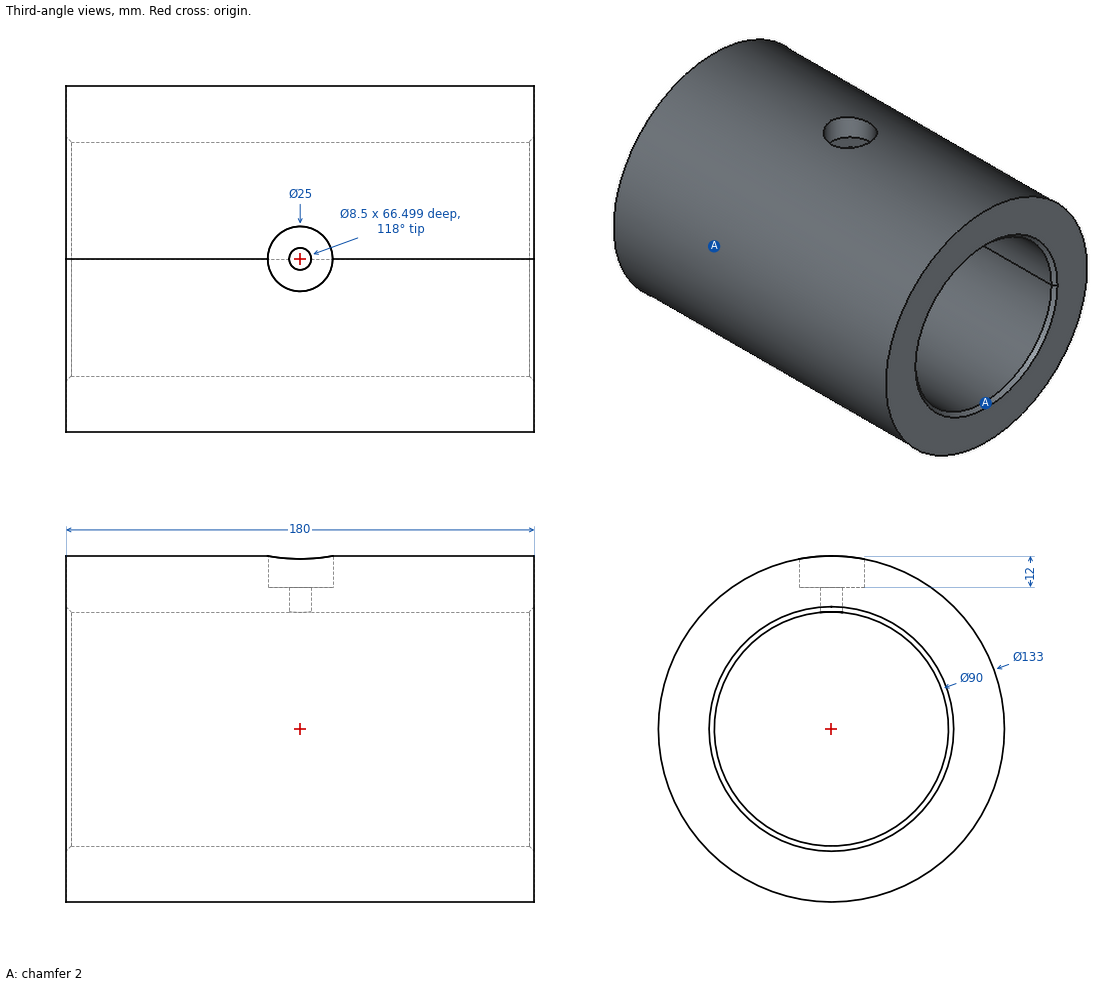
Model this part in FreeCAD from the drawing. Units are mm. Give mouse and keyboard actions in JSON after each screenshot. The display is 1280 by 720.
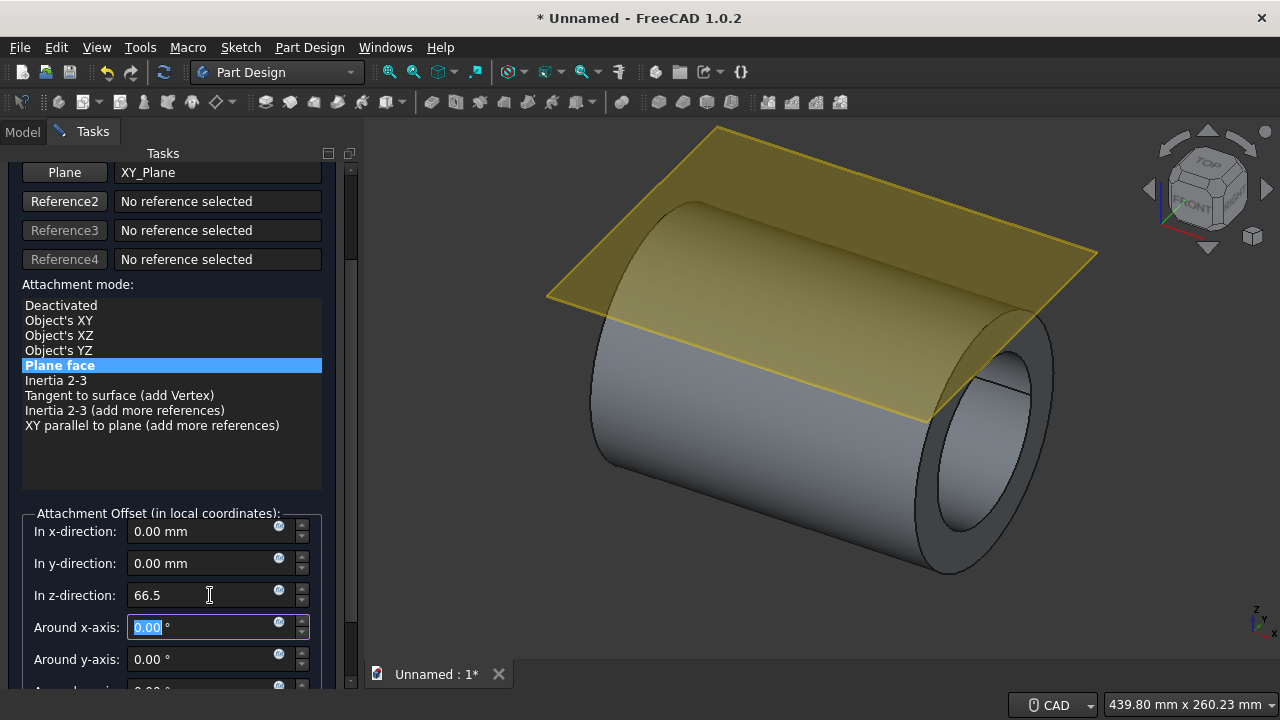
{"action": "scroll", "coordinate": [351, 426], "scroll_direction": "up", "scroll_amount": 3}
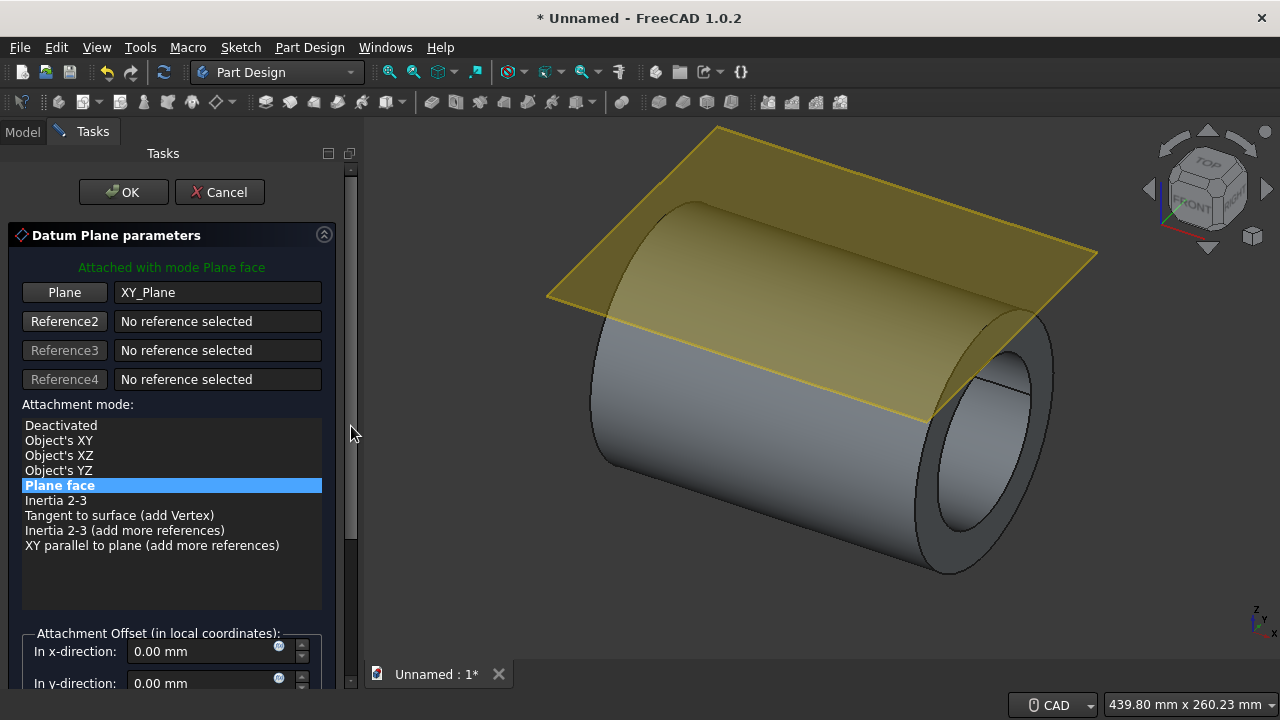
{"action": "left_click", "coordinate": [124, 192]}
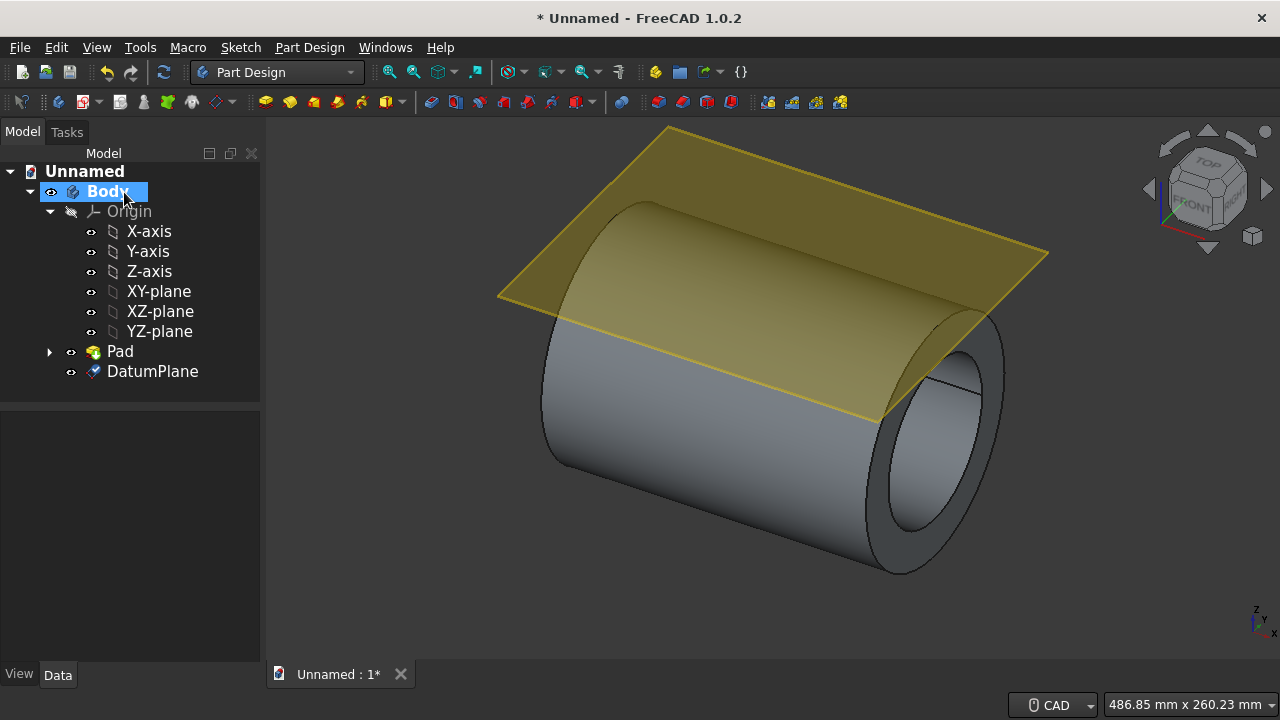
{"action": "left_click", "coordinate": [116, 372]}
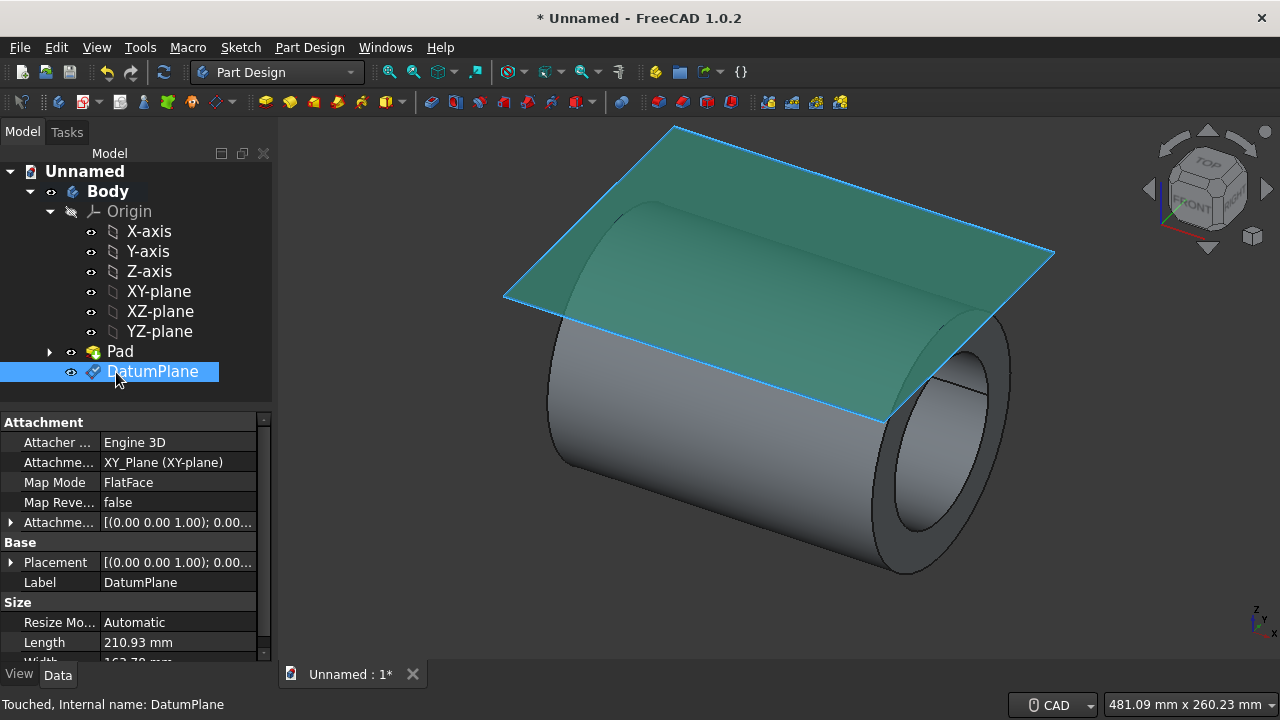
{"action": "left_click", "coordinate": [84, 102]}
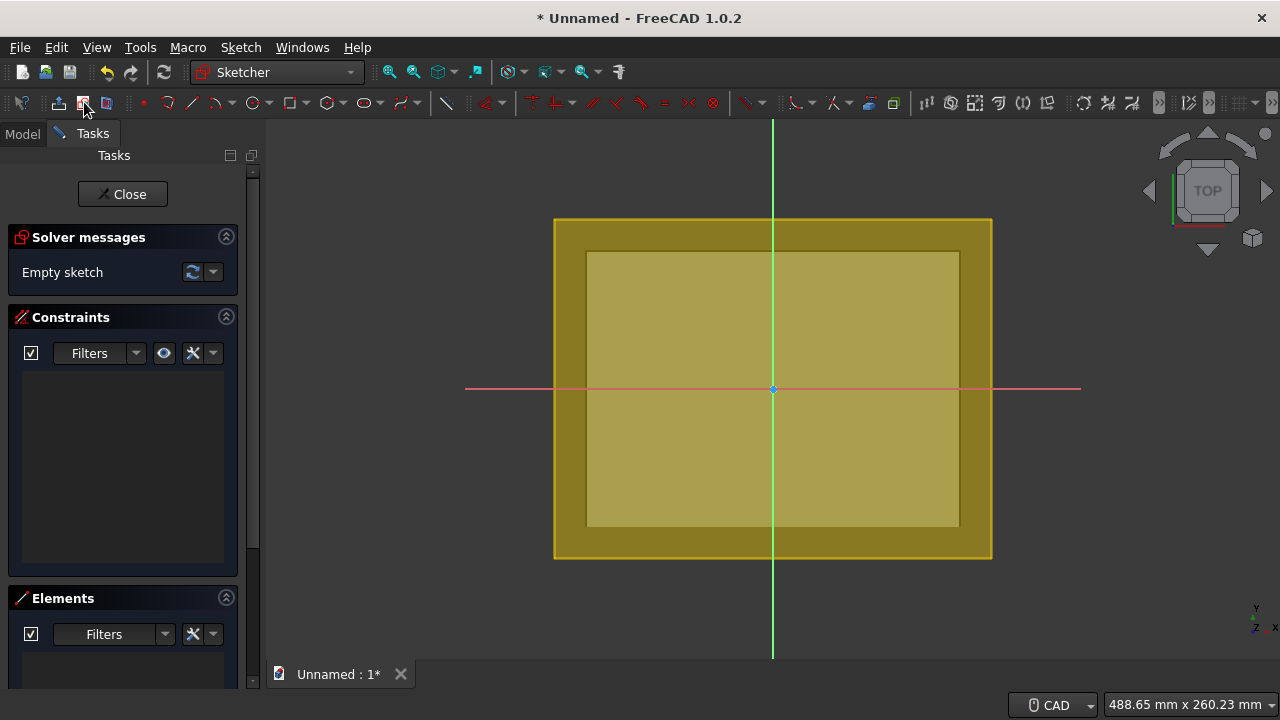
{"action": "scroll", "coordinate": [777, 389], "scroll_direction": "up", "scroll_amount": 15}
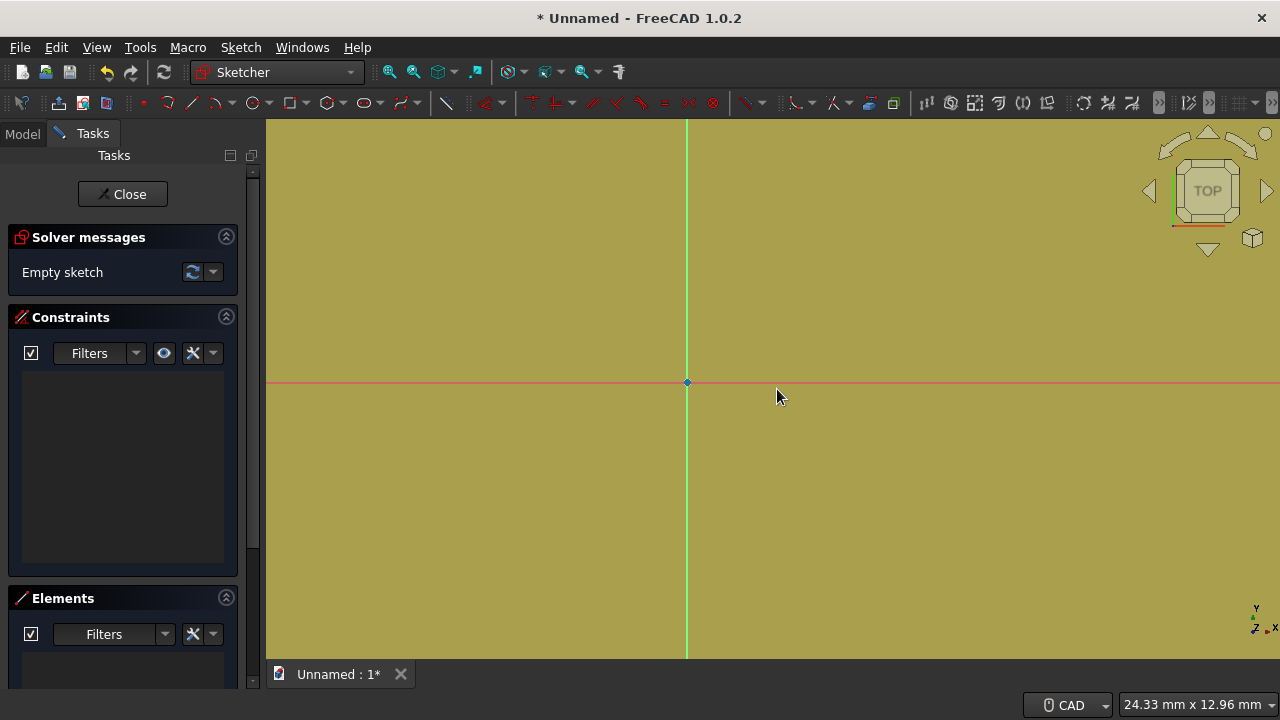
{"action": "left_click", "coordinate": [254, 104]}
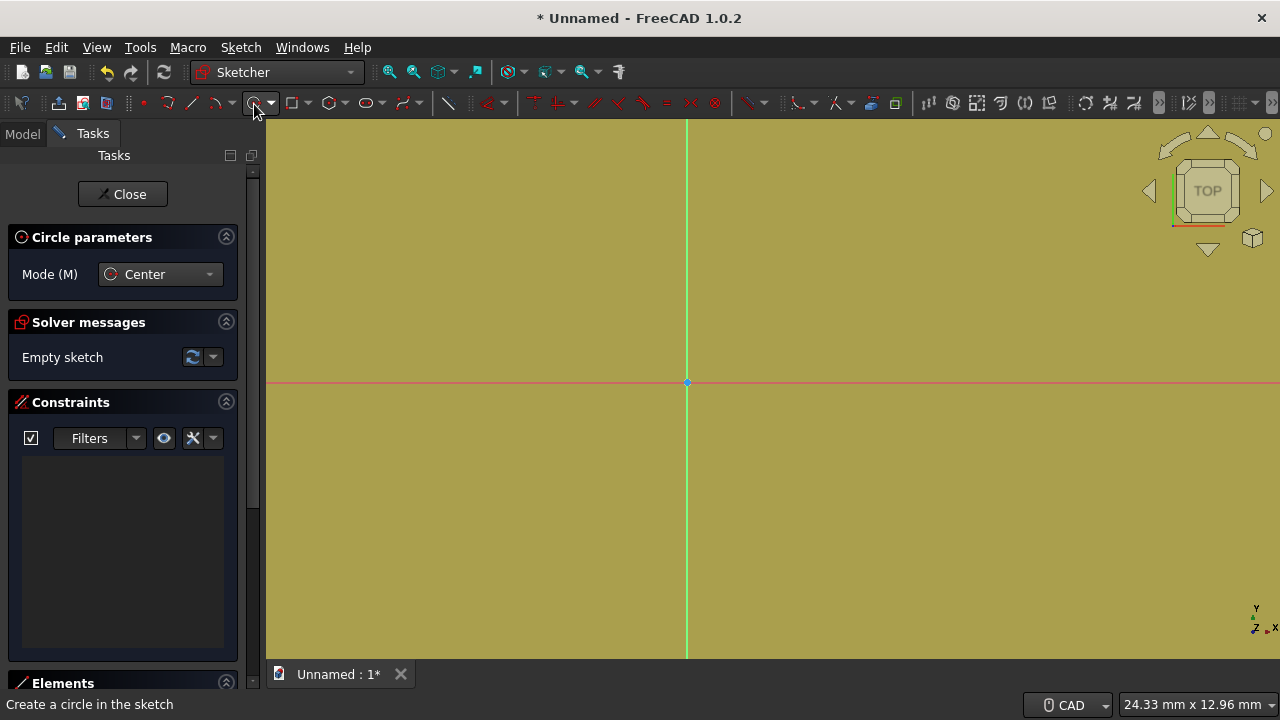
{"action": "left_click", "coordinate": [687, 383]}
{"action": "mouse_move", "coordinate": [812, 257]}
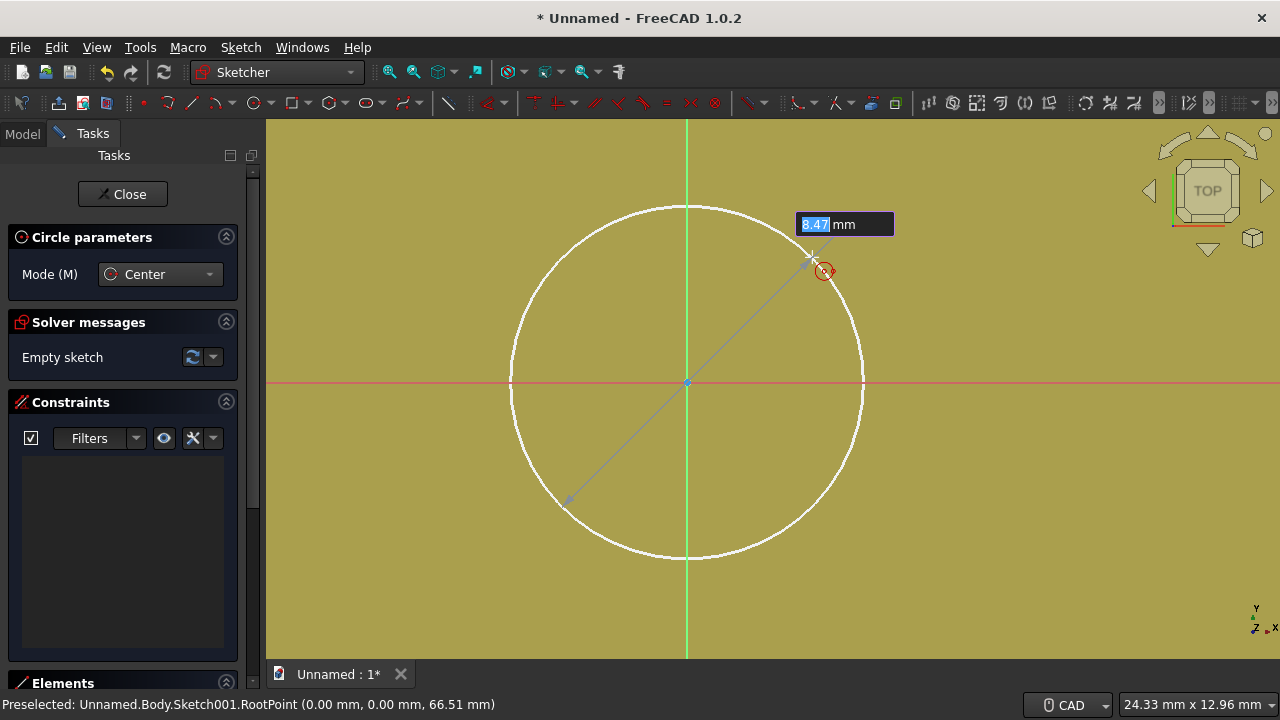
{"action": "type", "text": "8.5"}
{"action": "key", "text": "Return"}
{"action": "key", "text": "Escape"}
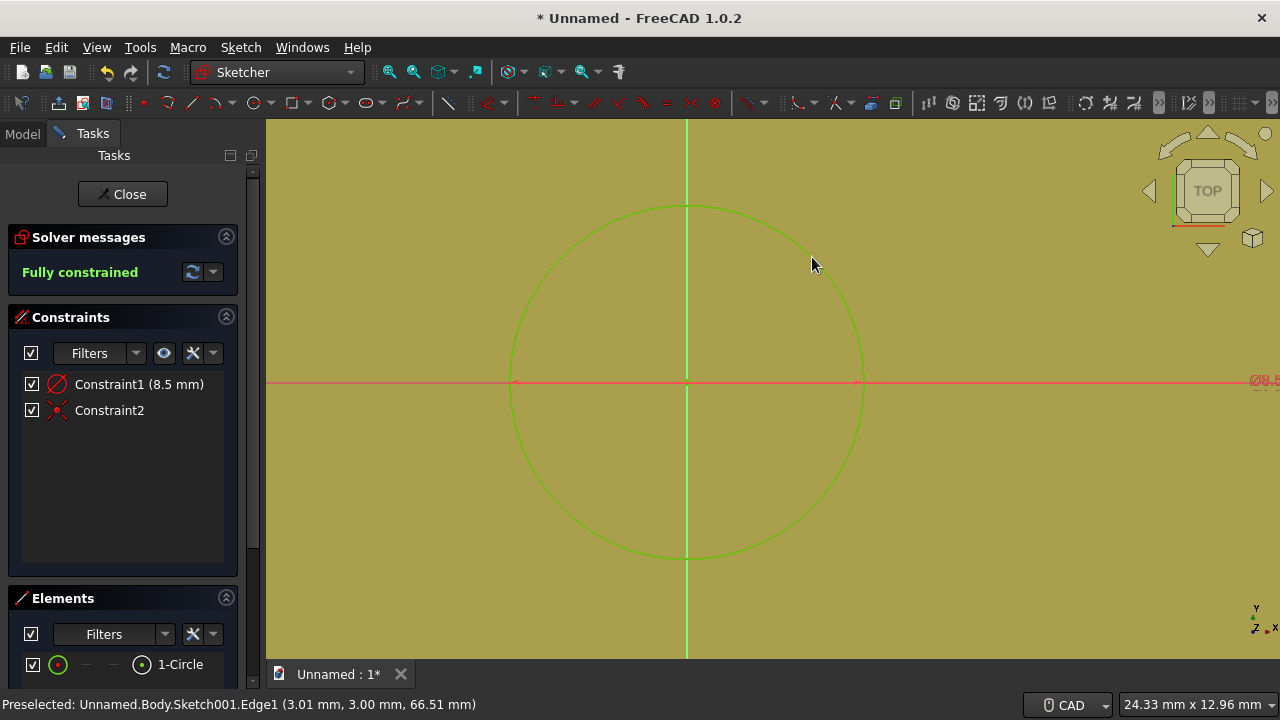
{"action": "left_click", "coordinate": [123, 194]}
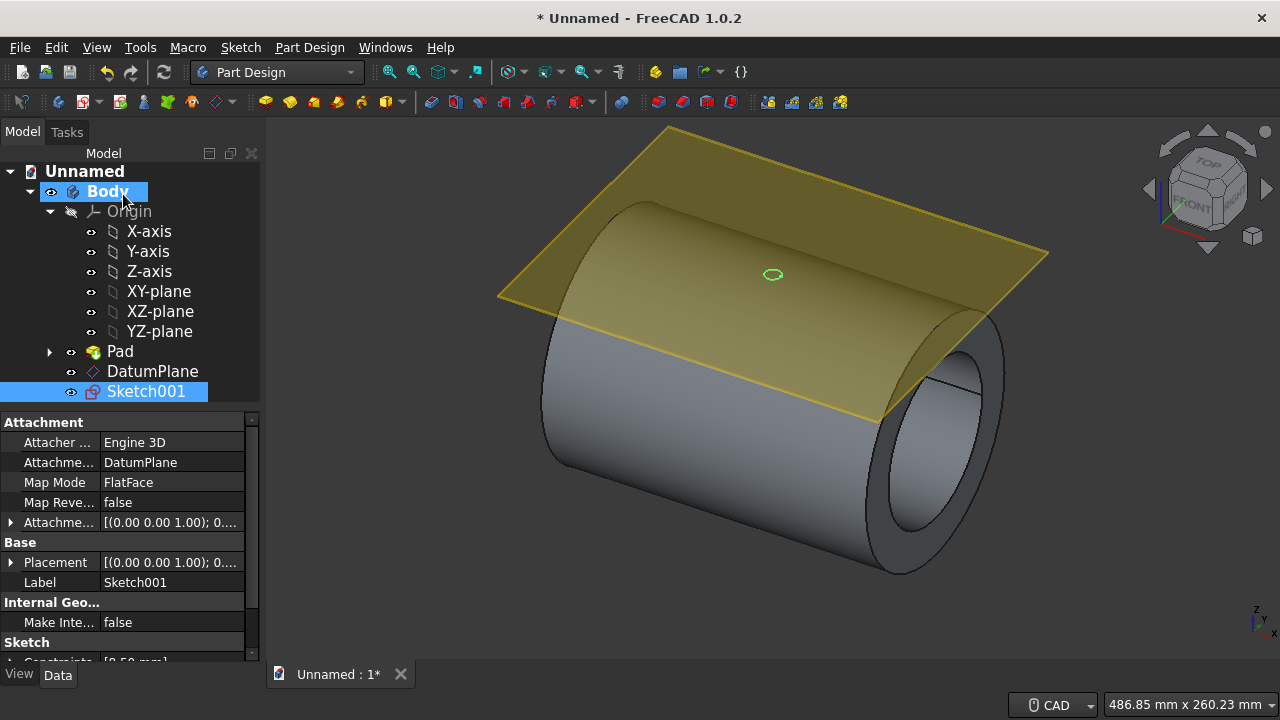
{"action": "left_click", "coordinate": [456, 102]}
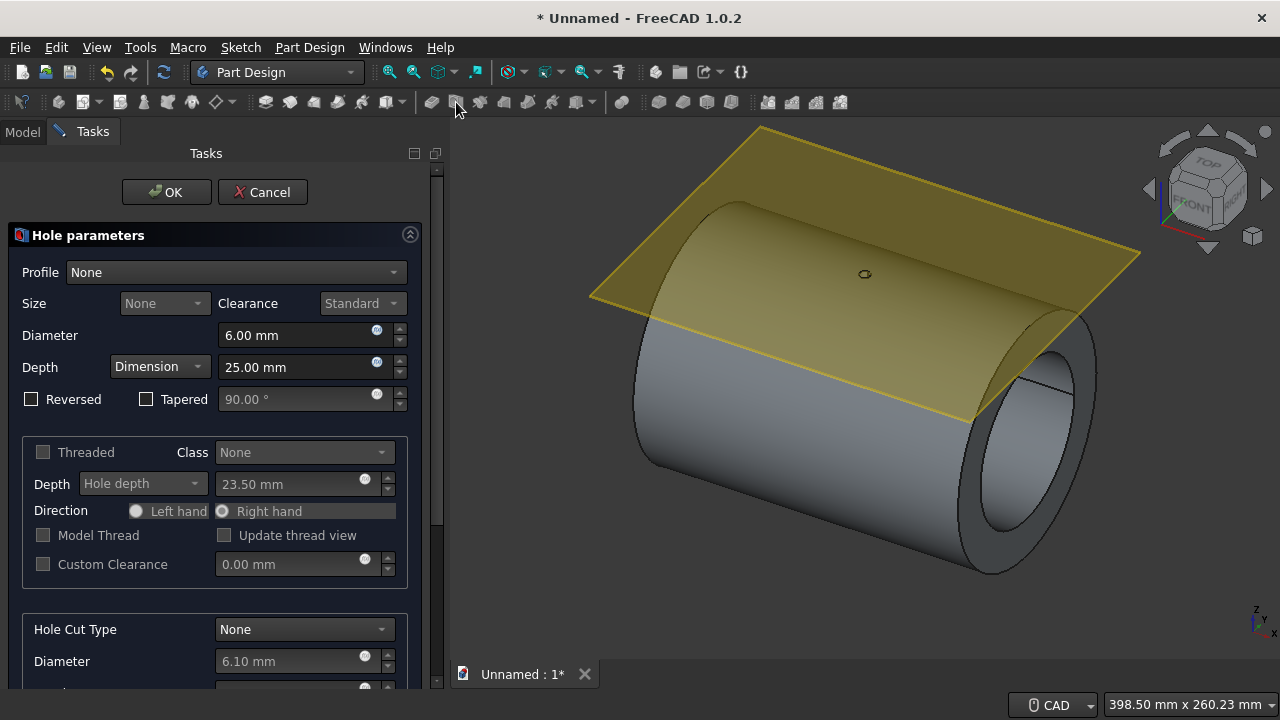
{"action": "triple_click", "coordinate": [305, 335]}